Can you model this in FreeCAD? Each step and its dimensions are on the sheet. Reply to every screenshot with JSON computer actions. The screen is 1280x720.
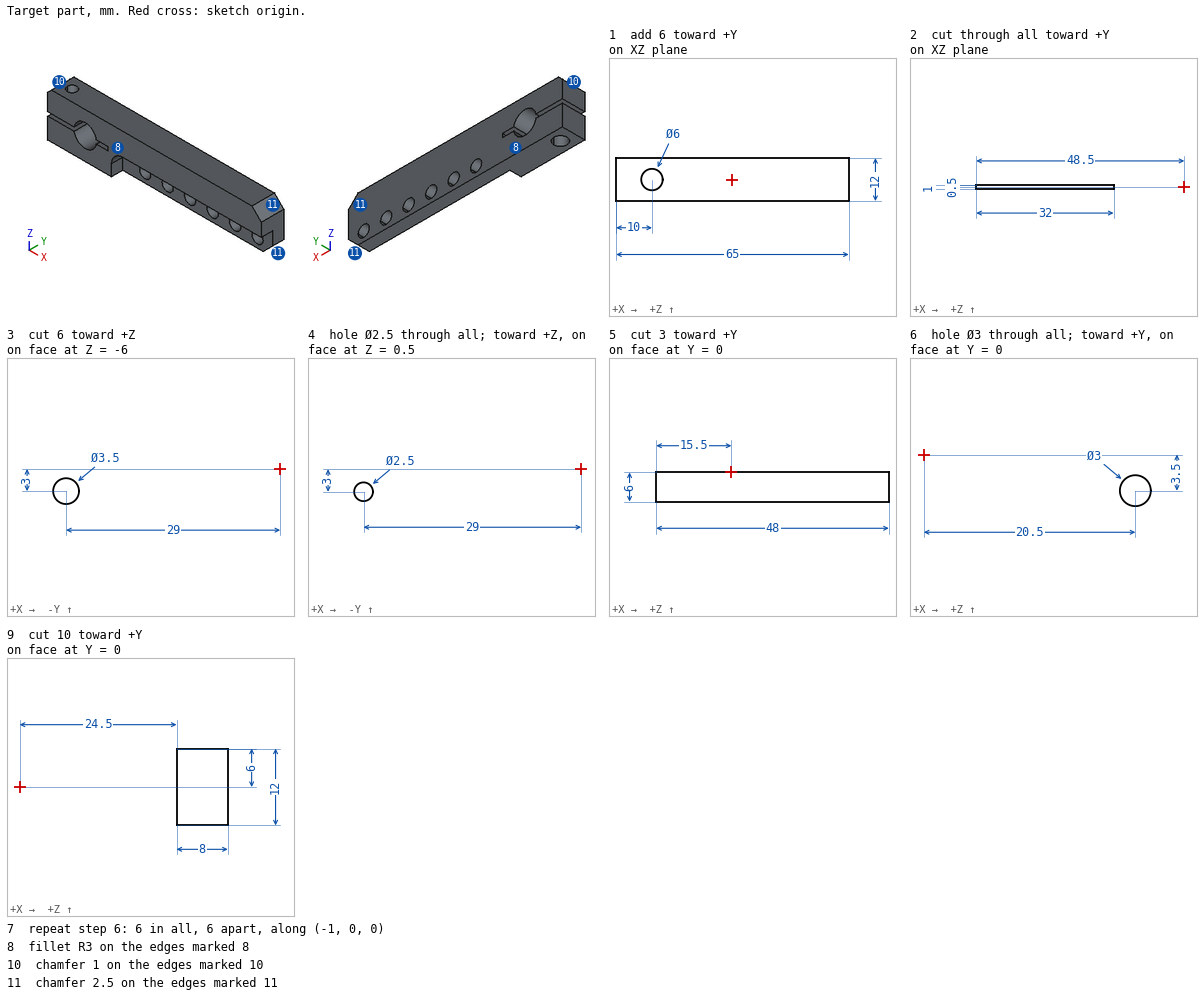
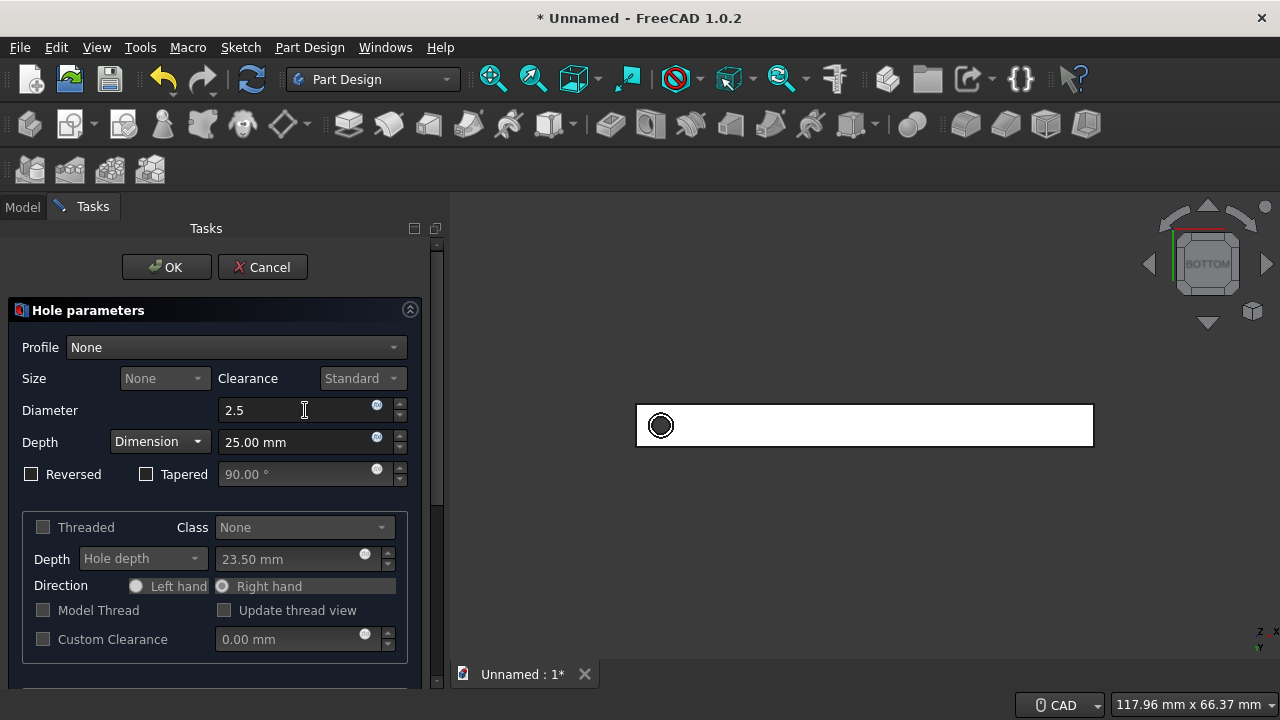
{"action": "left_click", "coordinate": [161, 442]}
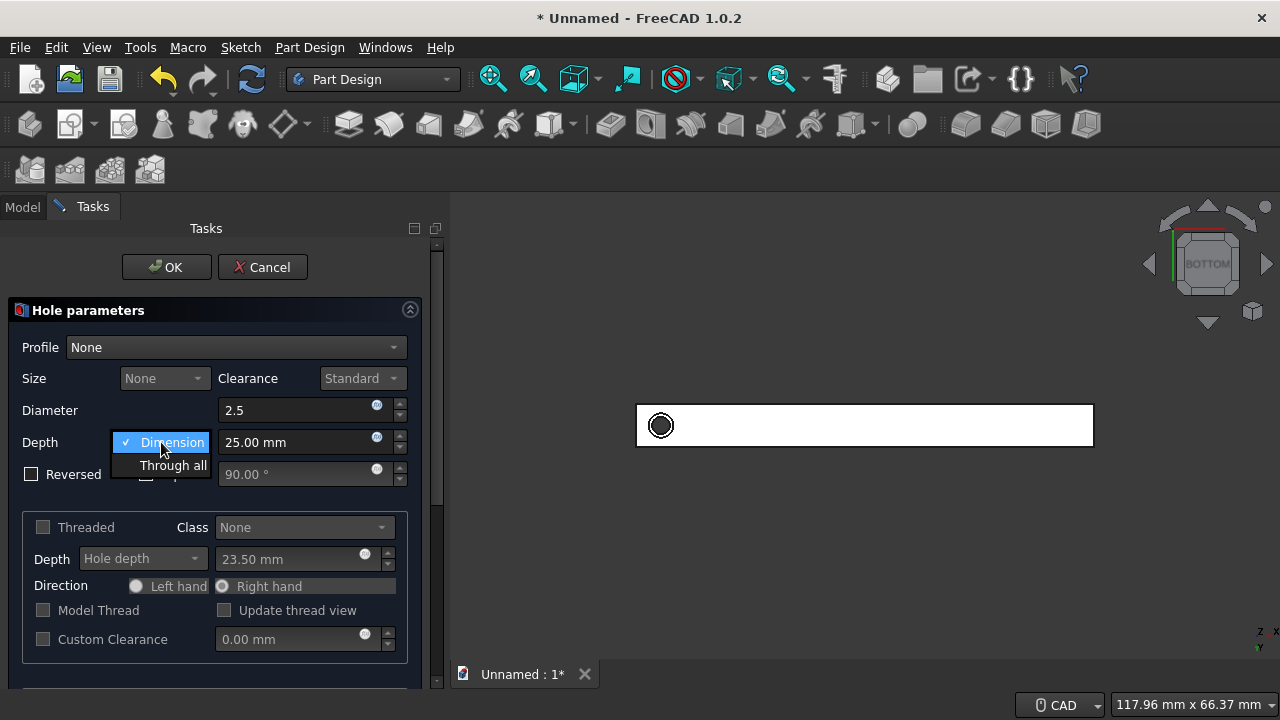
{"action": "left_click", "coordinate": [160, 466]}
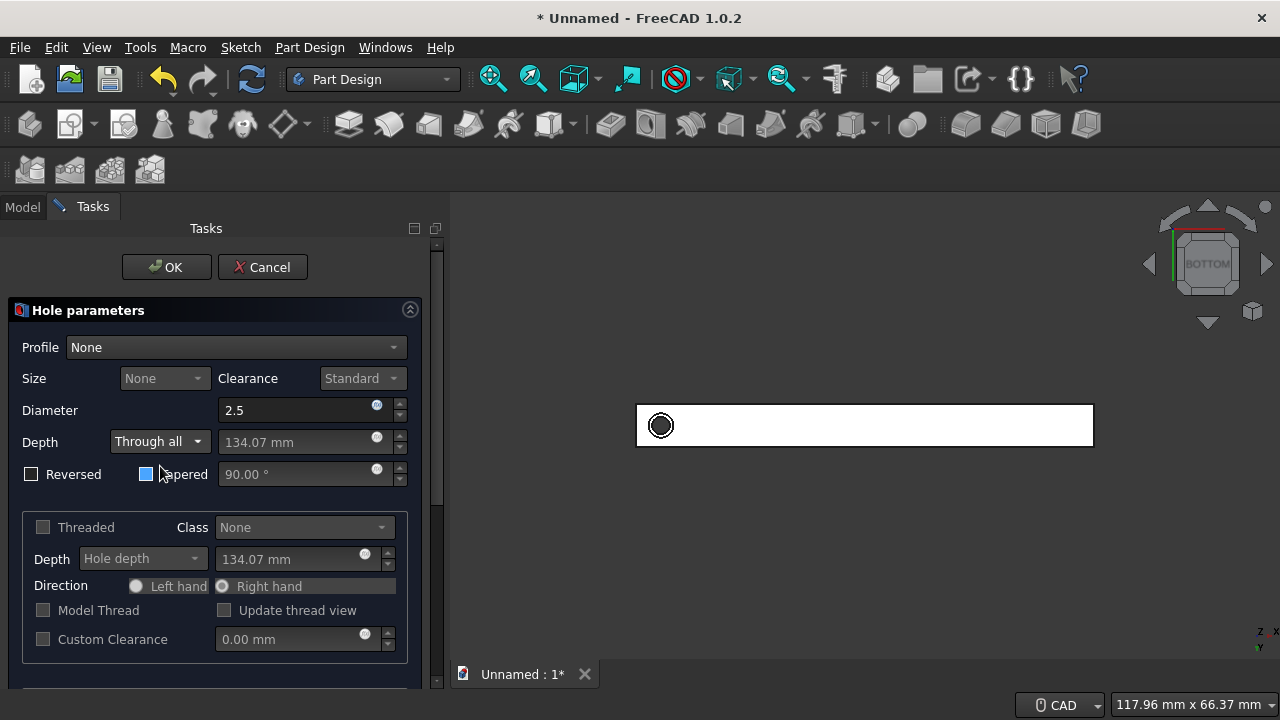
{"action": "left_click", "coordinate": [167, 267]}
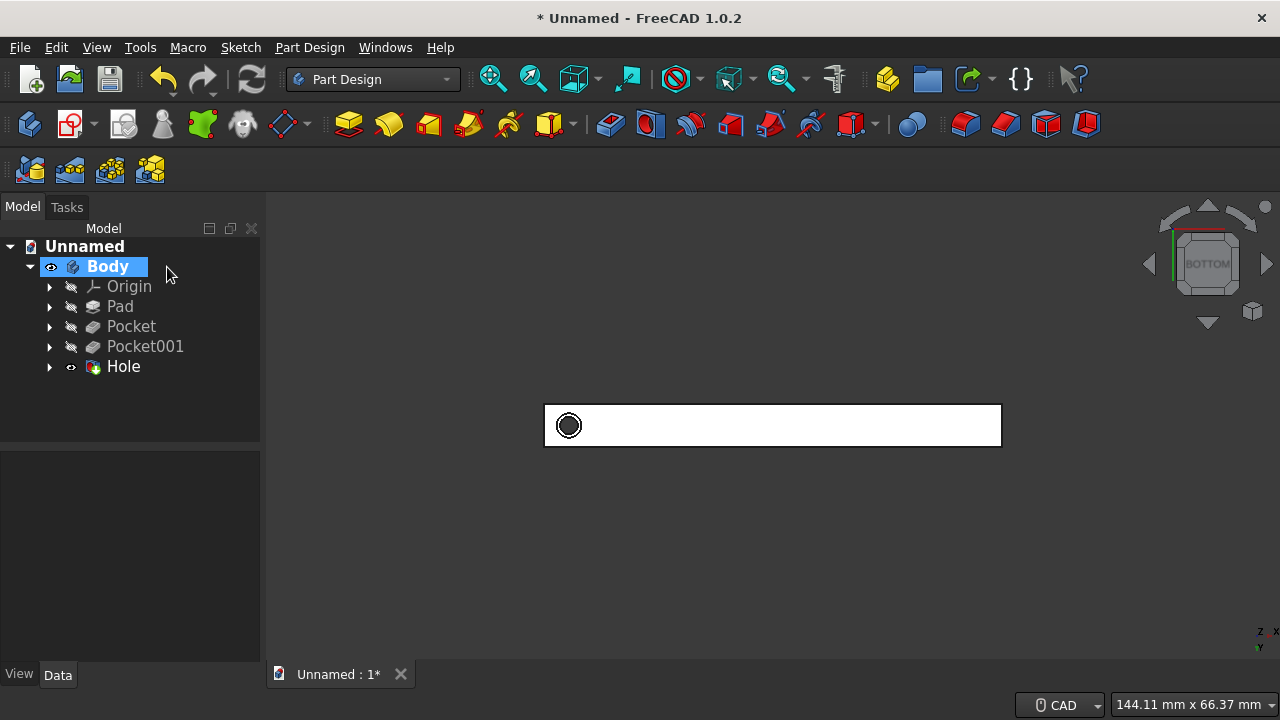
{"action": "key", "text": "0"}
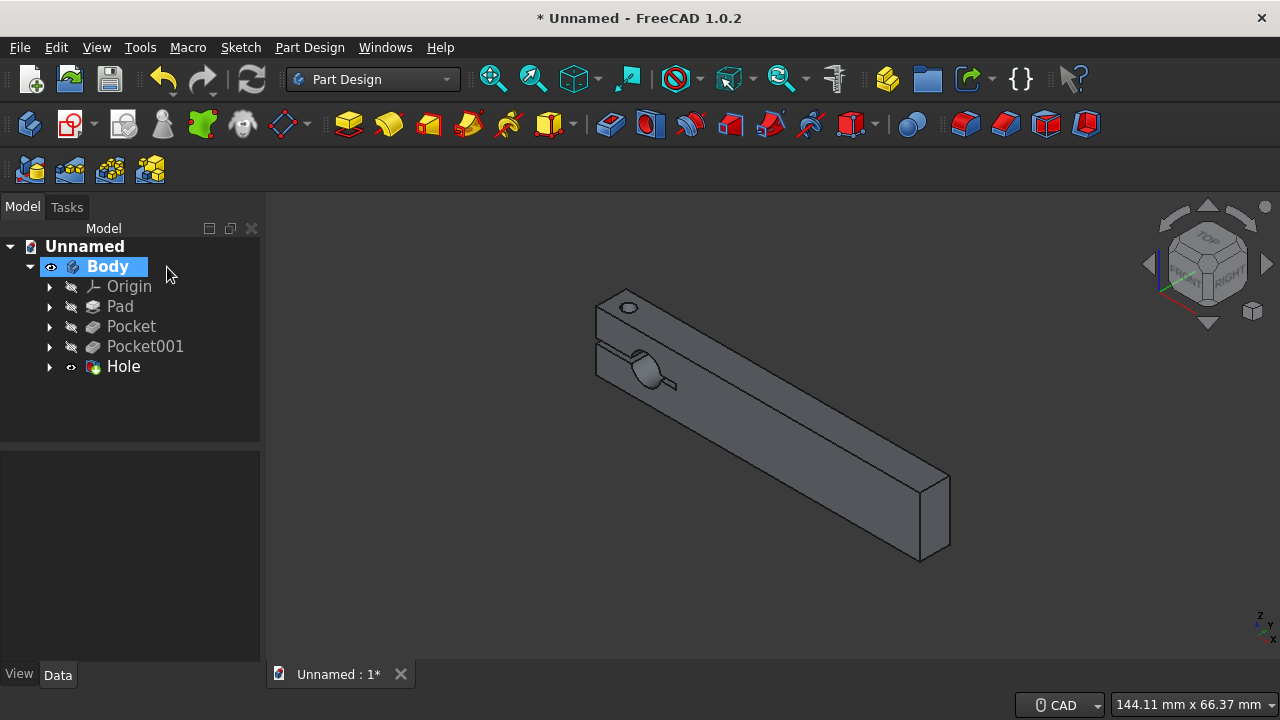
{"action": "left_click", "coordinate": [850, 486]}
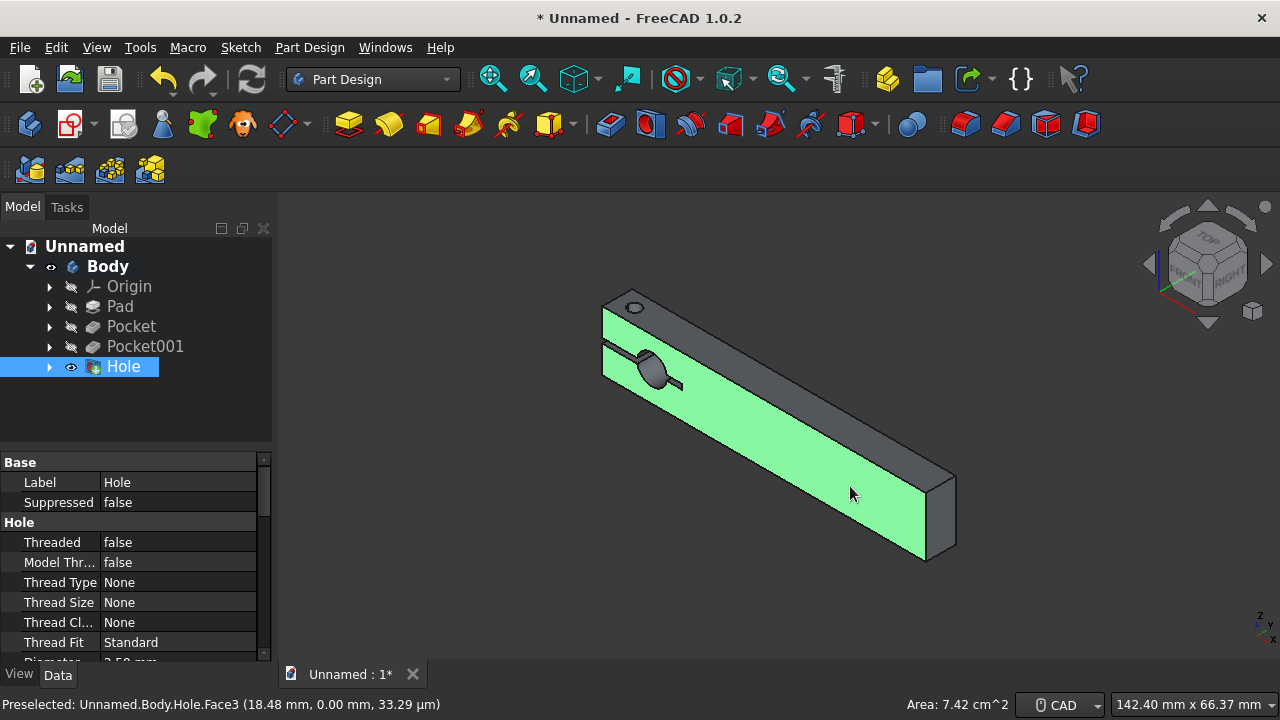
{"action": "left_click", "coordinate": [70, 124]}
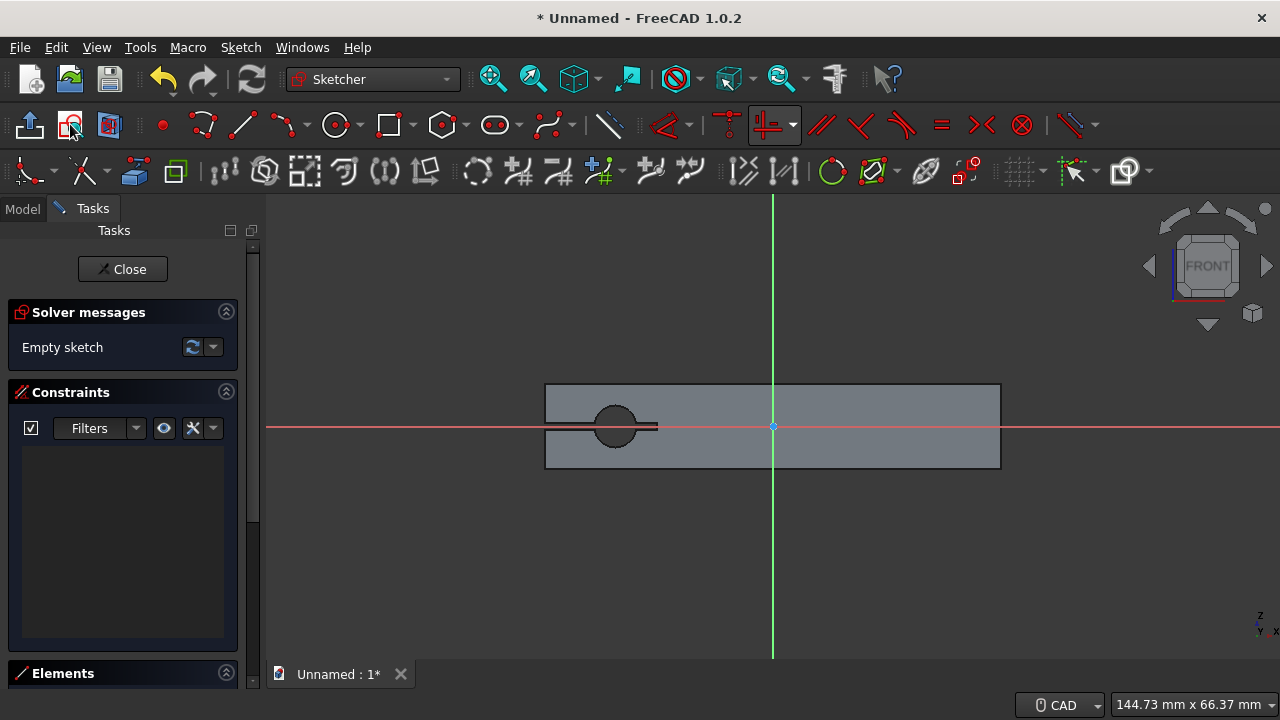
{"action": "scroll", "coordinate": [988, 473], "scroll_direction": "up", "scroll_amount": 3}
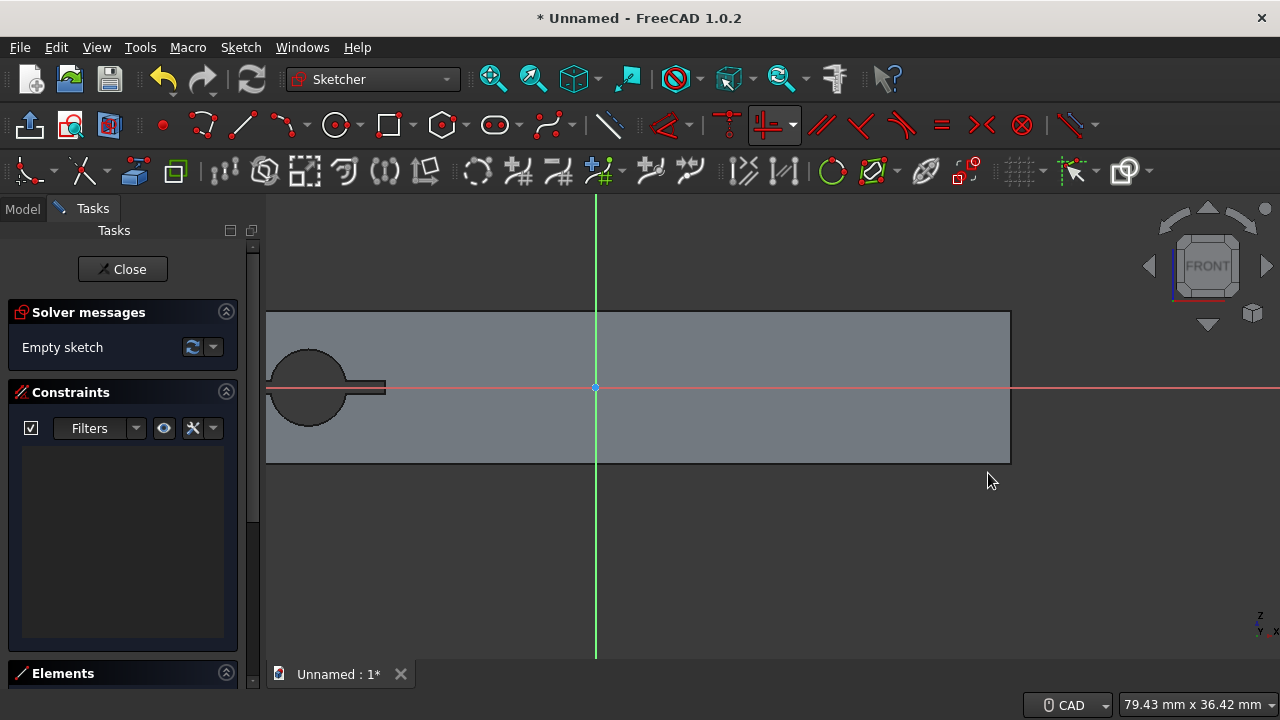
{"action": "left_click", "coordinate": [390, 126]}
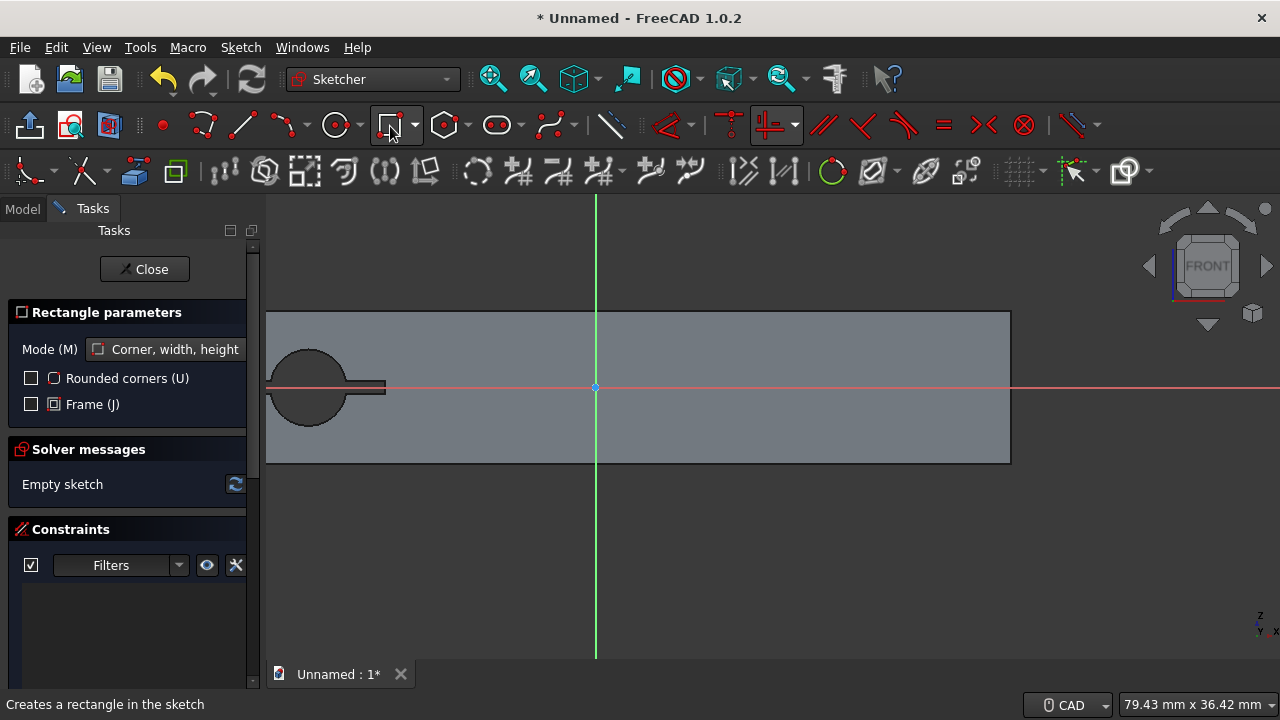
{"action": "left_click", "coordinate": [398, 388]}
{"action": "left_click", "coordinate": [1011, 464]}
{"action": "key", "text": "Escape"}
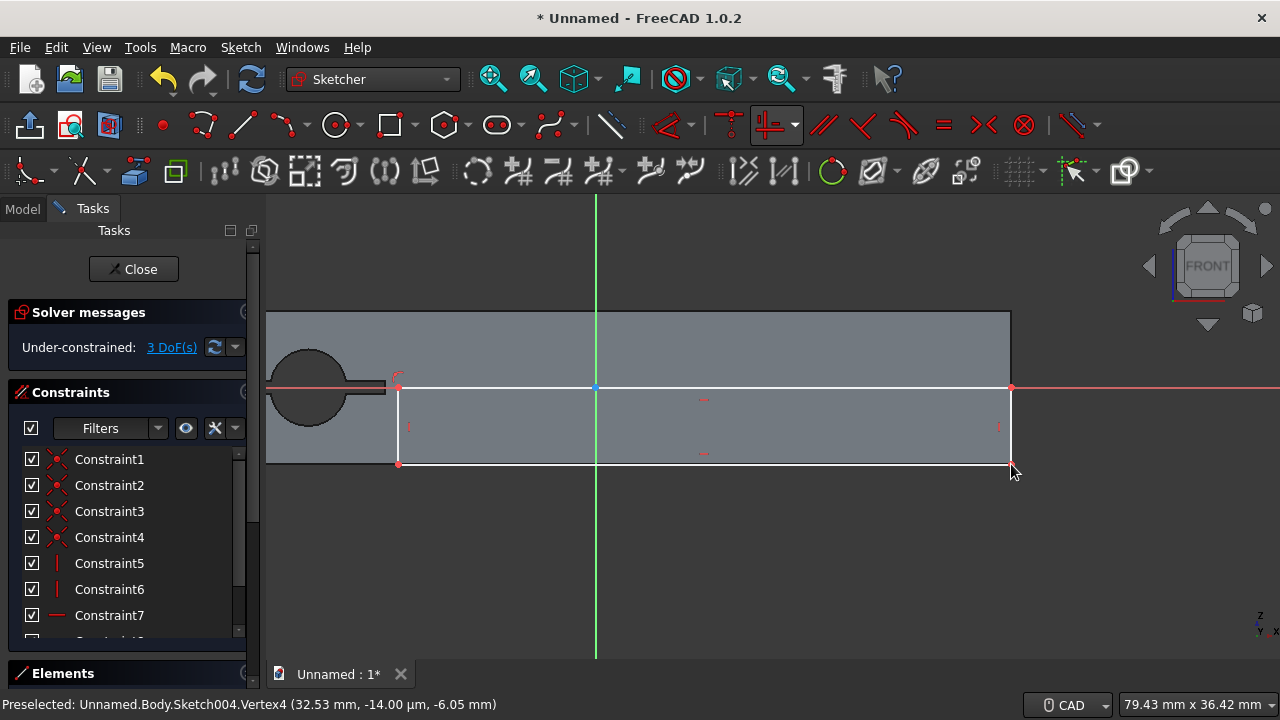
{"action": "key", "text": "d"}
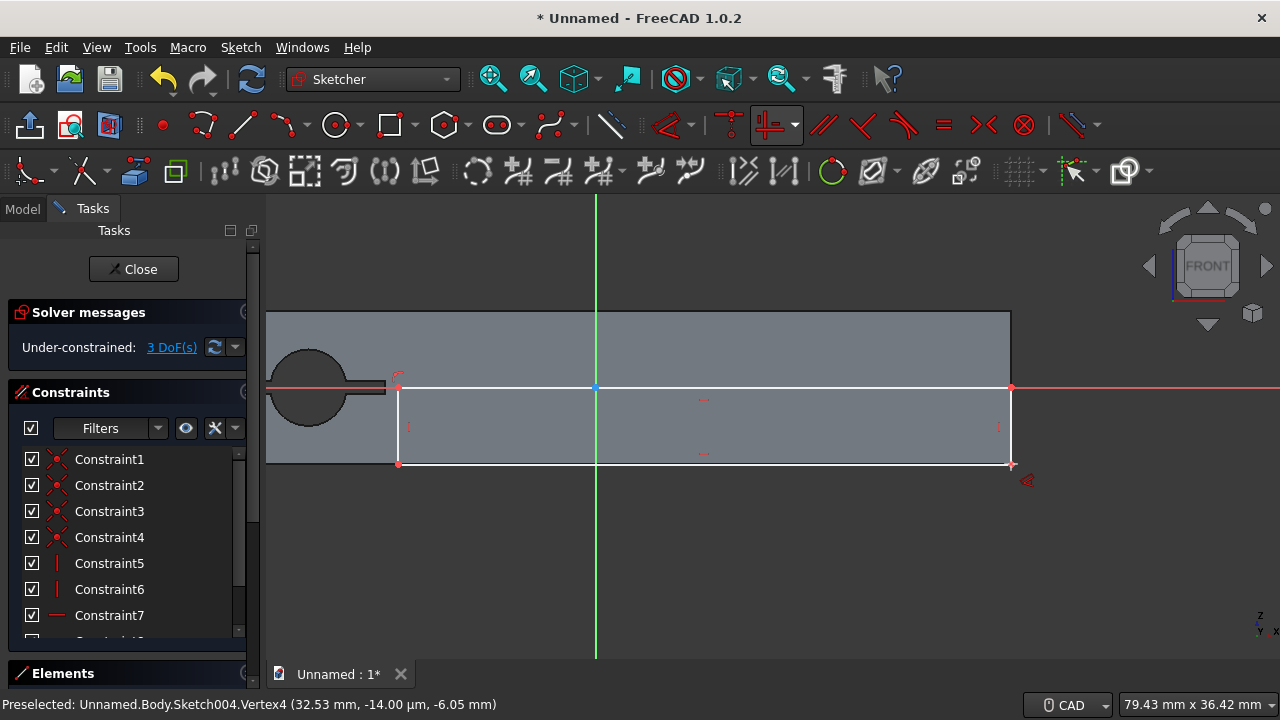
{"action": "left_click", "coordinate": [398, 411]}
{"action": "left_click", "coordinate": [364, 426]}